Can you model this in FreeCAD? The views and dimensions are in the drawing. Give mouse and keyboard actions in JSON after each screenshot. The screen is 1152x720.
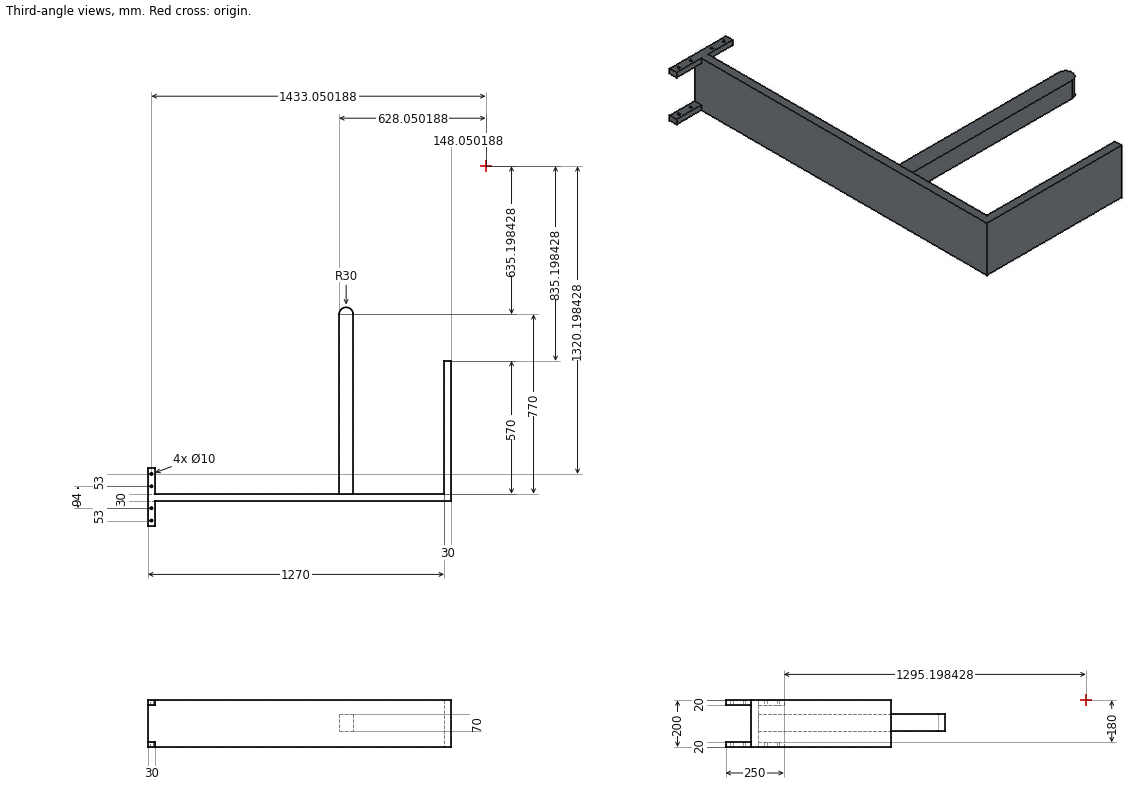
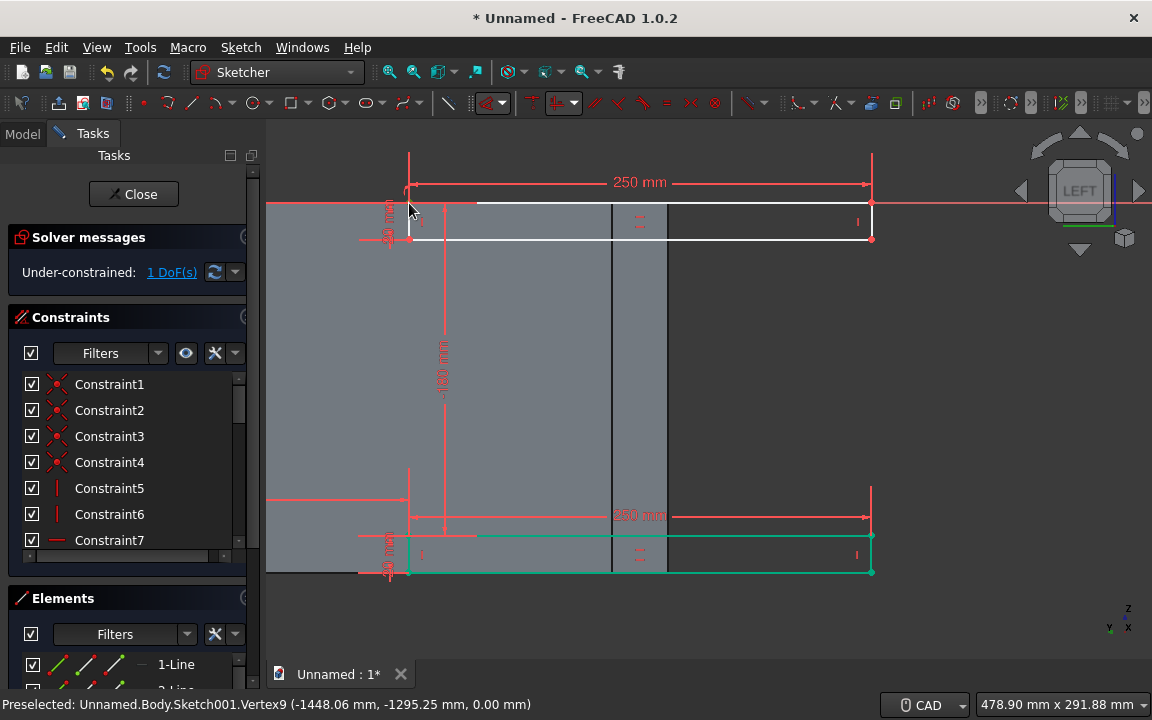
{"action": "key", "text": "l"}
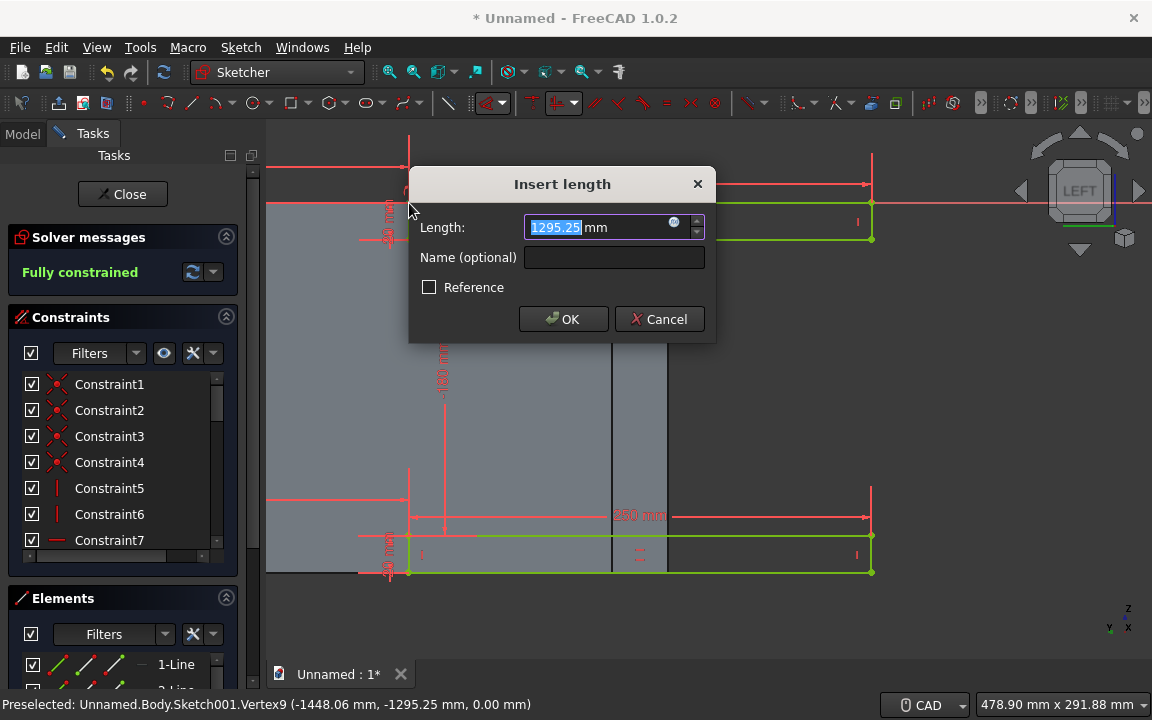
{"action": "type", "text": "1295.198428"}
{"action": "key", "text": "Return"}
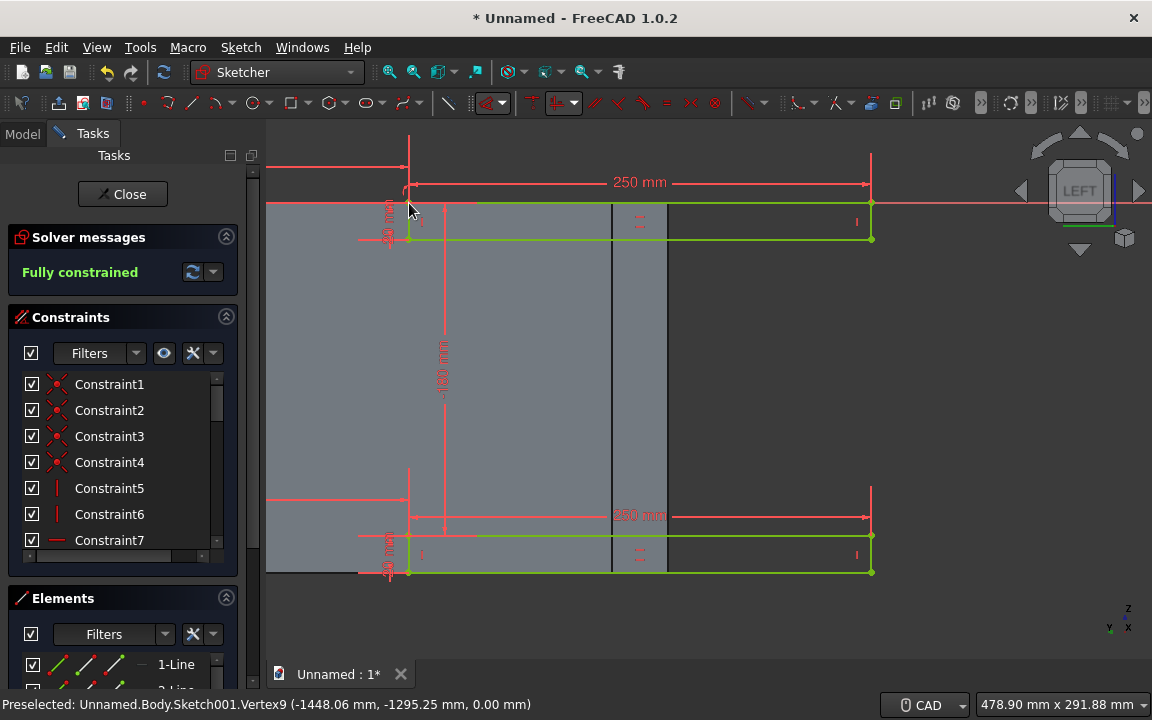
{"action": "left_click", "coordinate": [123, 194]}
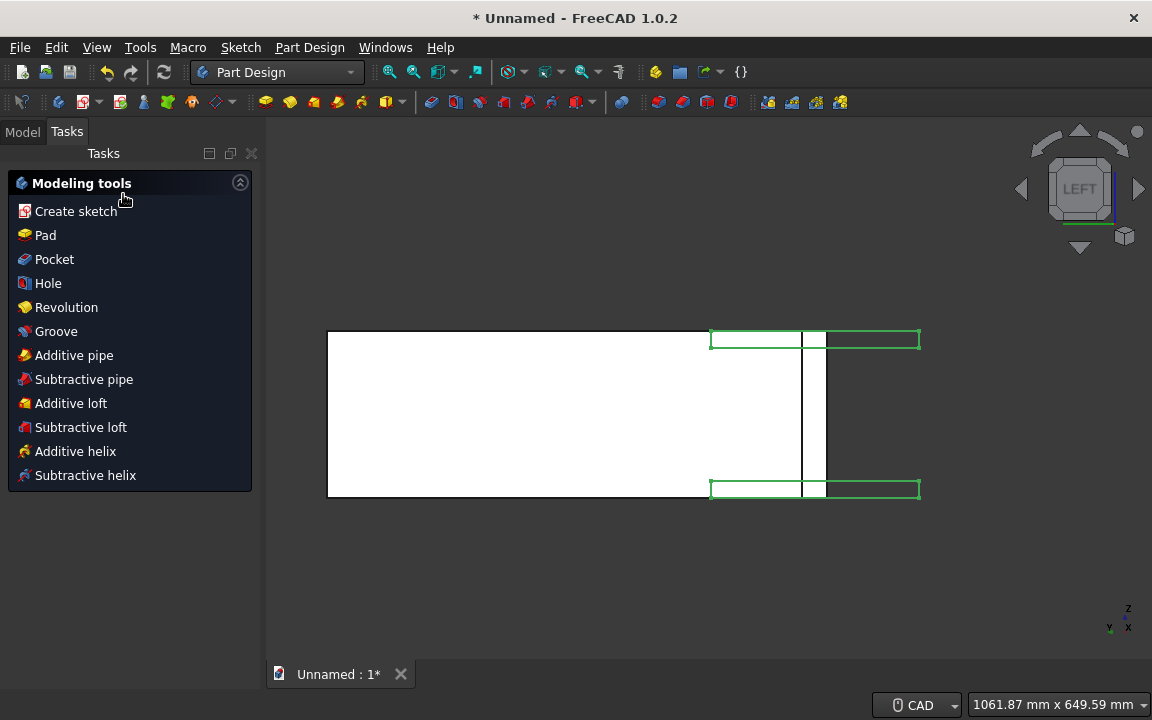
{"action": "left_click", "coordinate": [266, 102]}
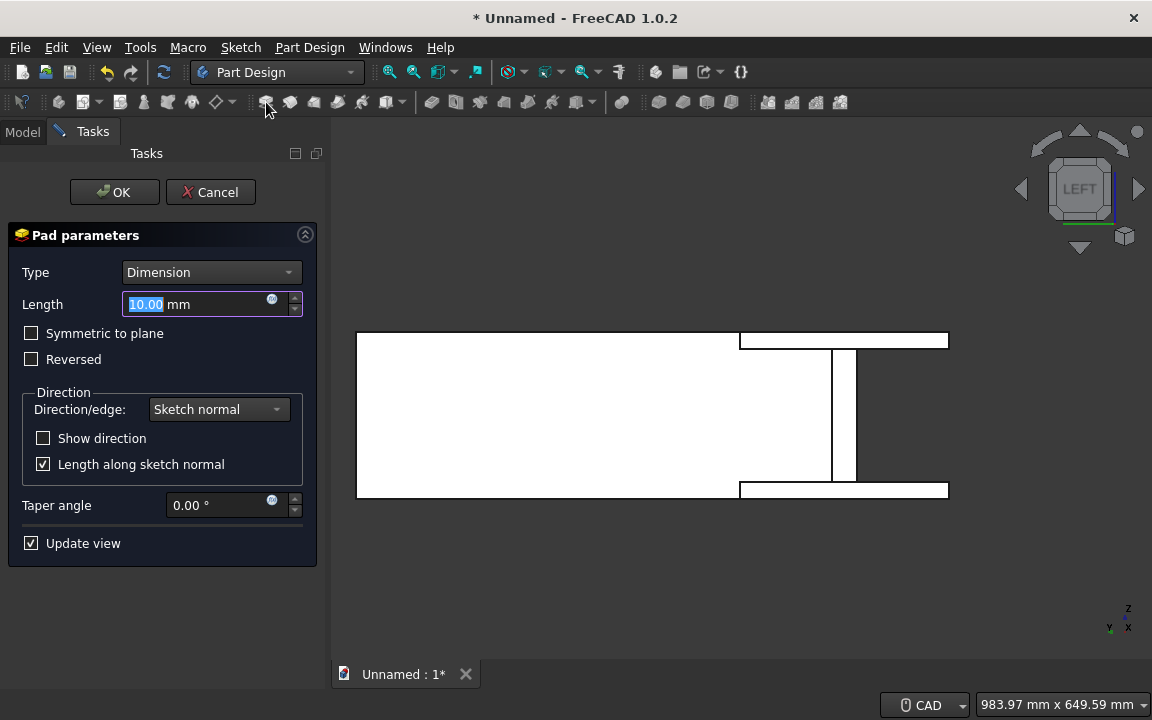
{"action": "type", "text": "30"}
{"action": "key", "text": "Tab"}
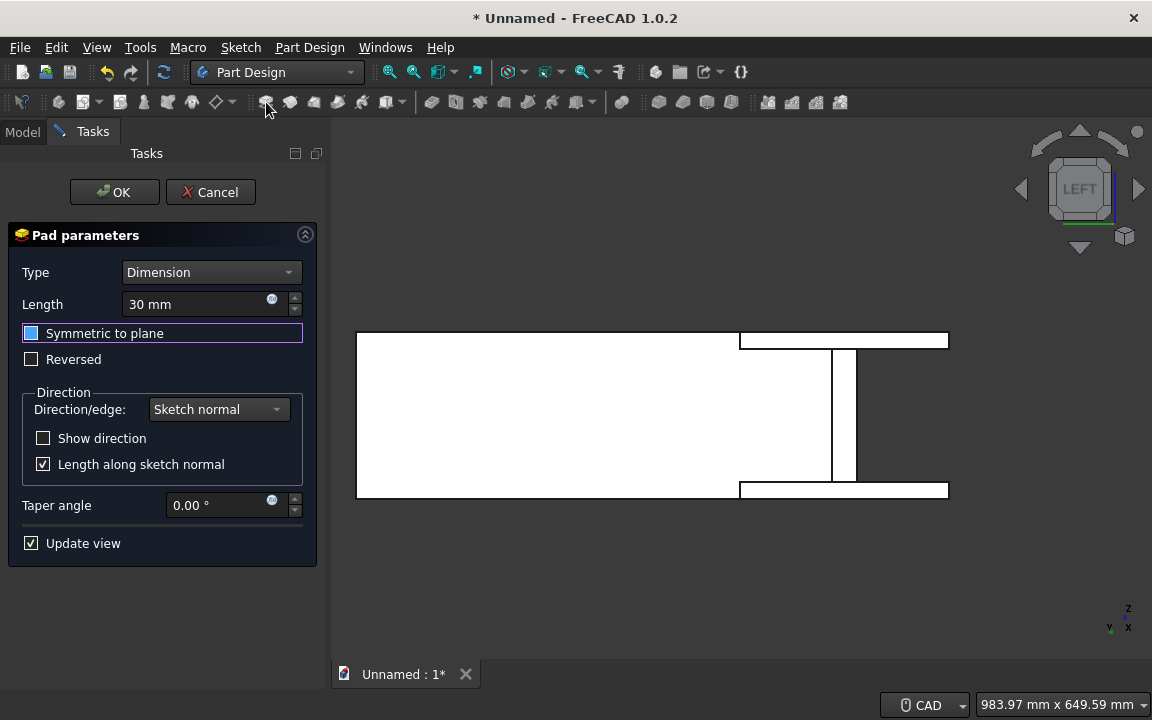
{"action": "left_click", "coordinate": [30, 359]}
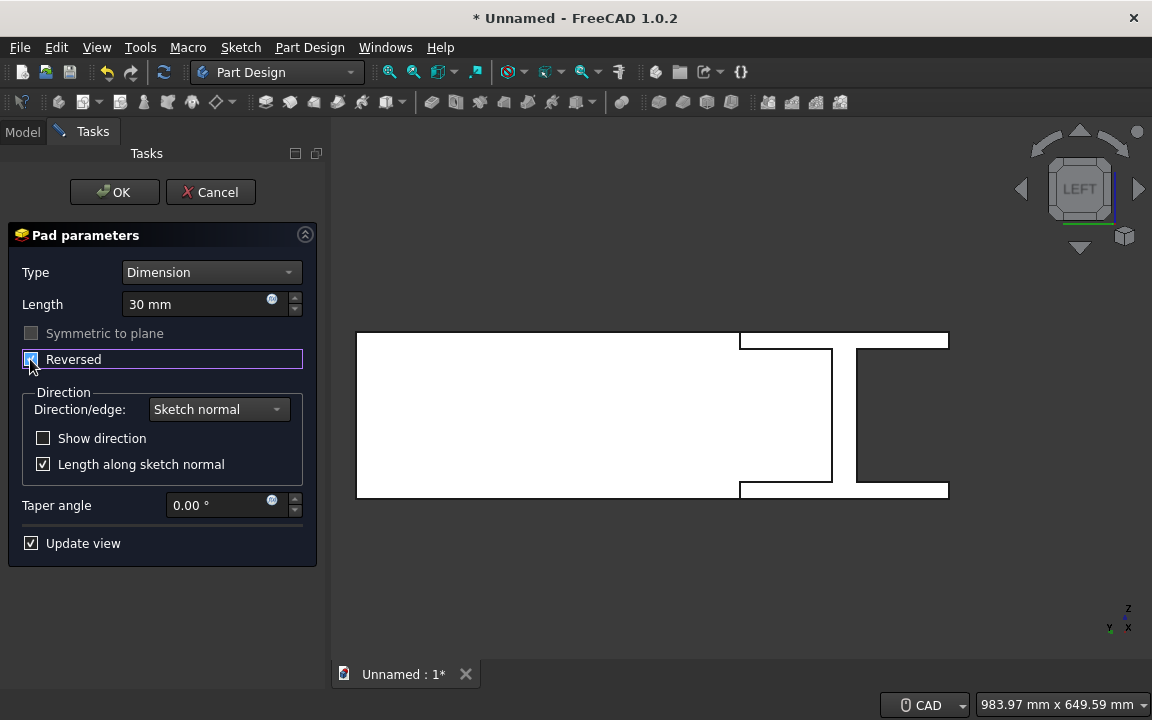
{"action": "left_click", "coordinate": [115, 192]}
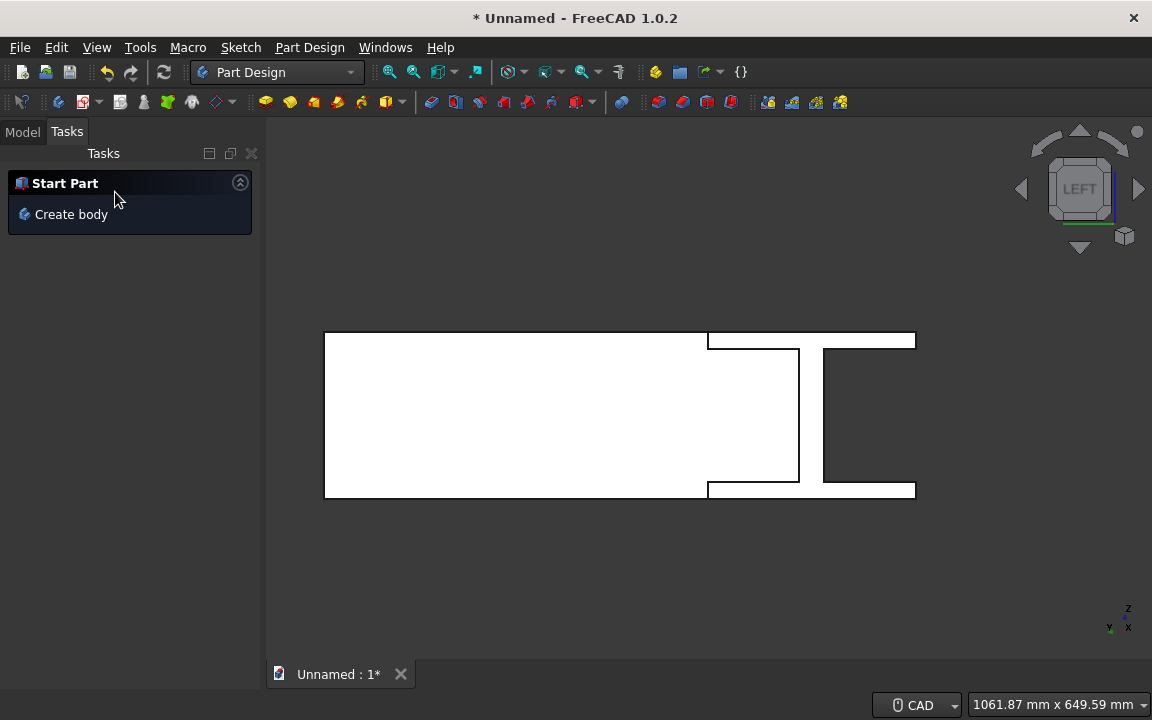
{"action": "key", "text": "5"}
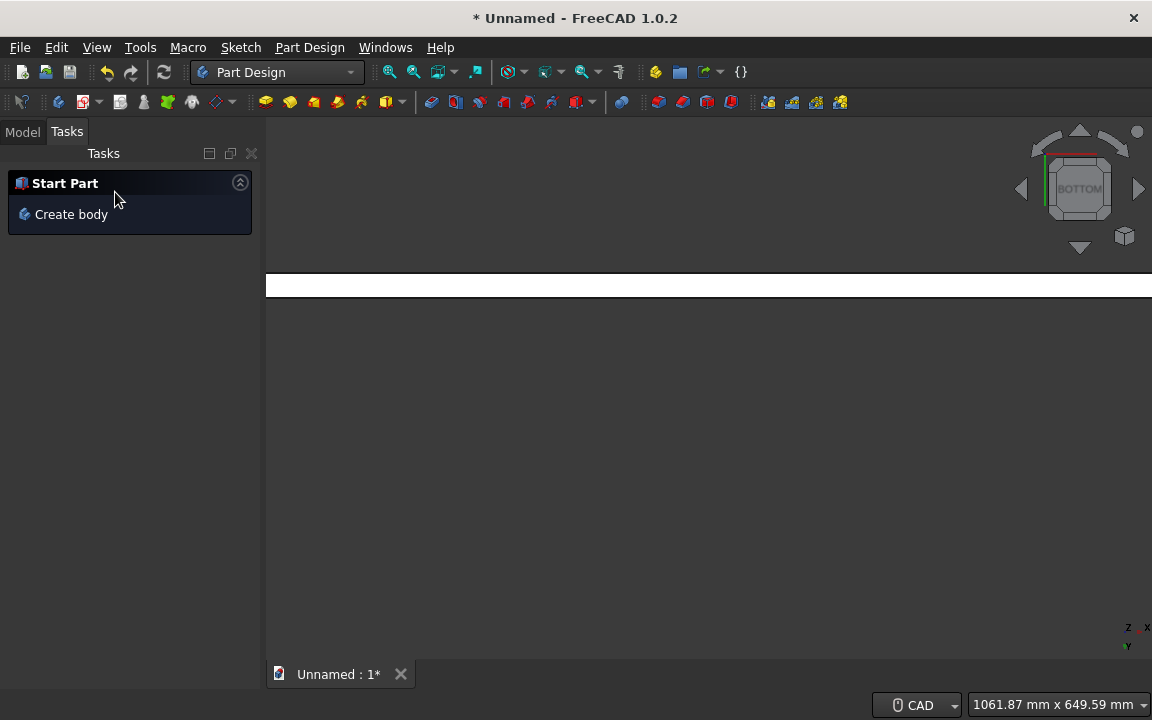
{"action": "left_click", "coordinate": [390, 72]}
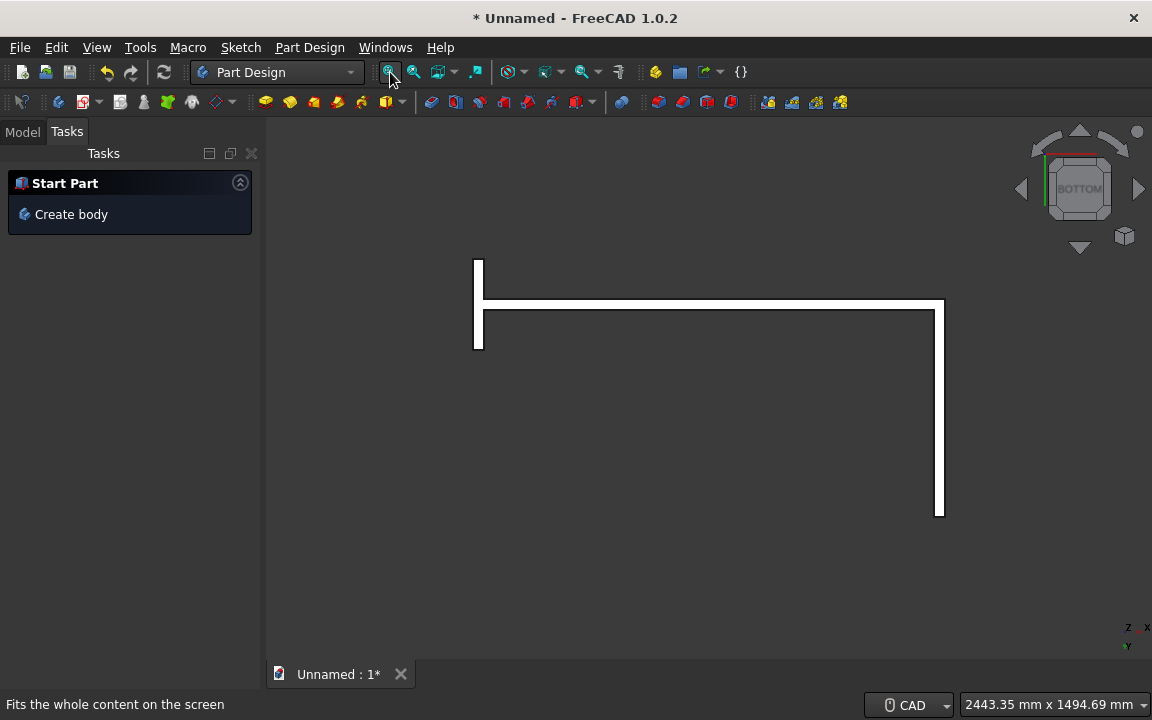
{"action": "scroll", "coordinate": [634, 305], "scroll_direction": "up", "scroll_amount": 6}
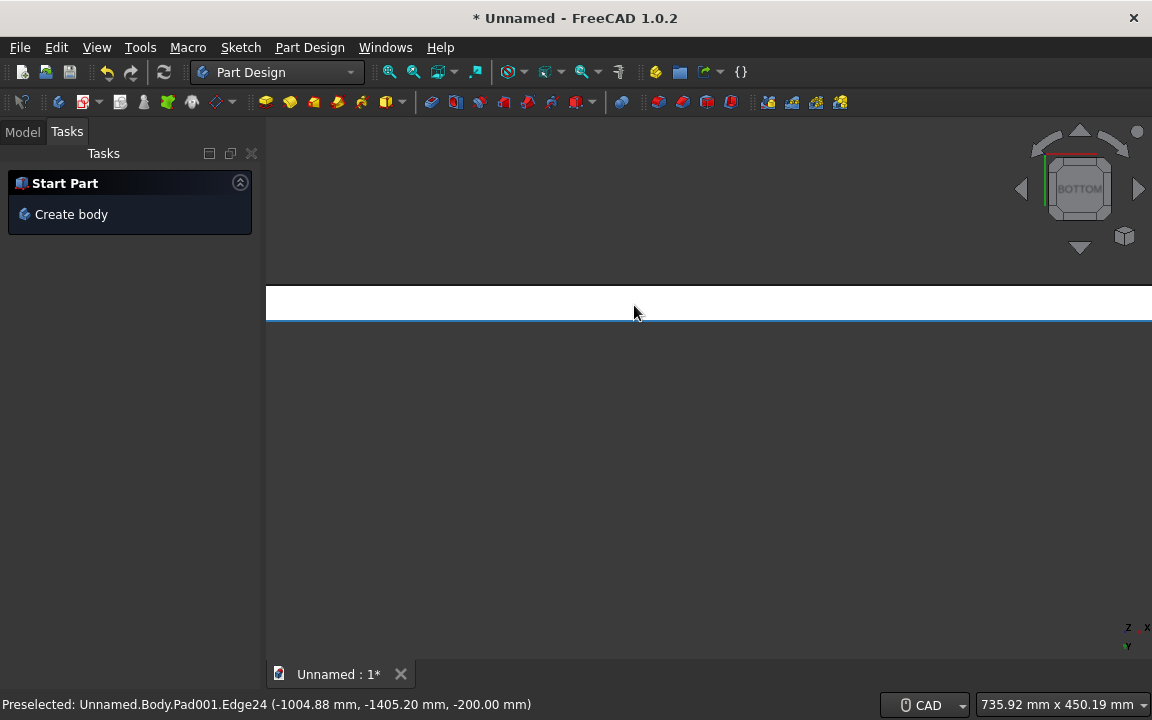
{"action": "left_click", "coordinate": [633, 308]}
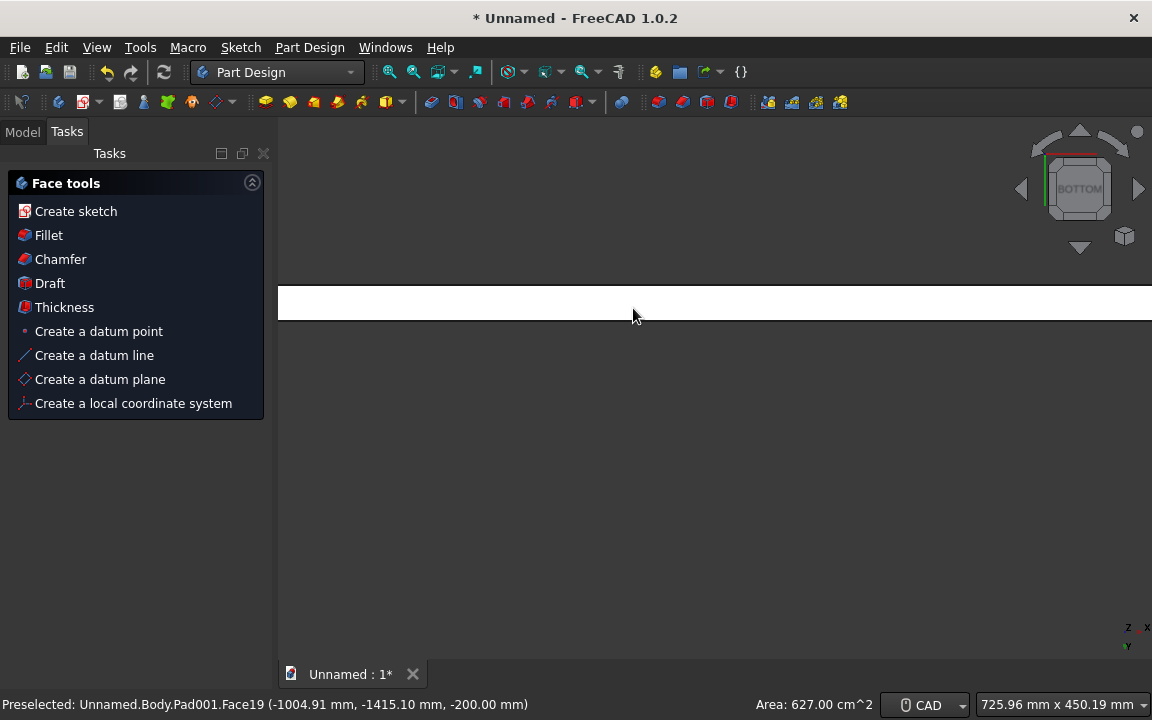
{"action": "left_click", "coordinate": [84, 102]}